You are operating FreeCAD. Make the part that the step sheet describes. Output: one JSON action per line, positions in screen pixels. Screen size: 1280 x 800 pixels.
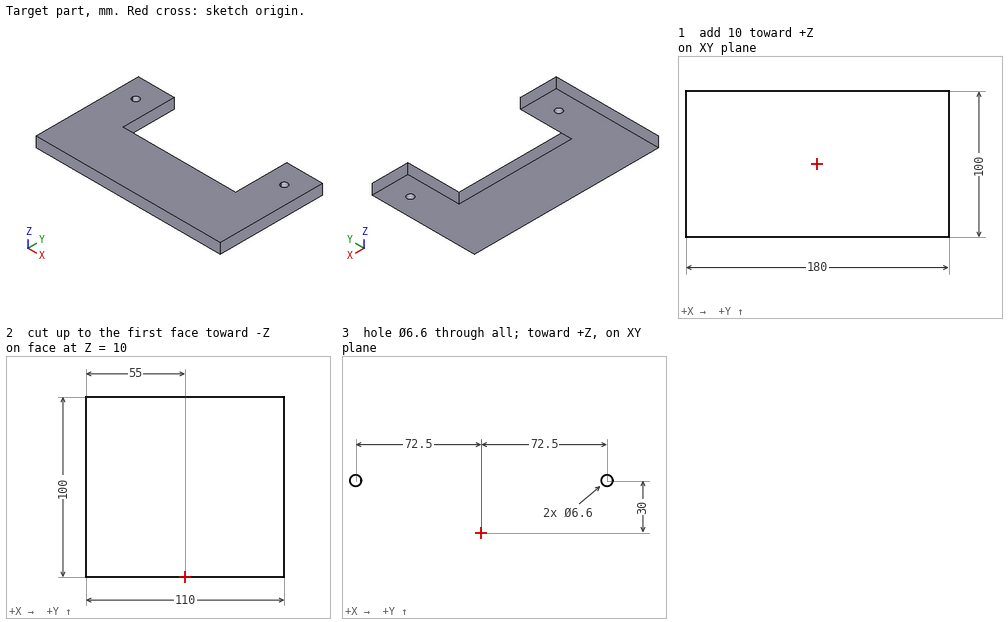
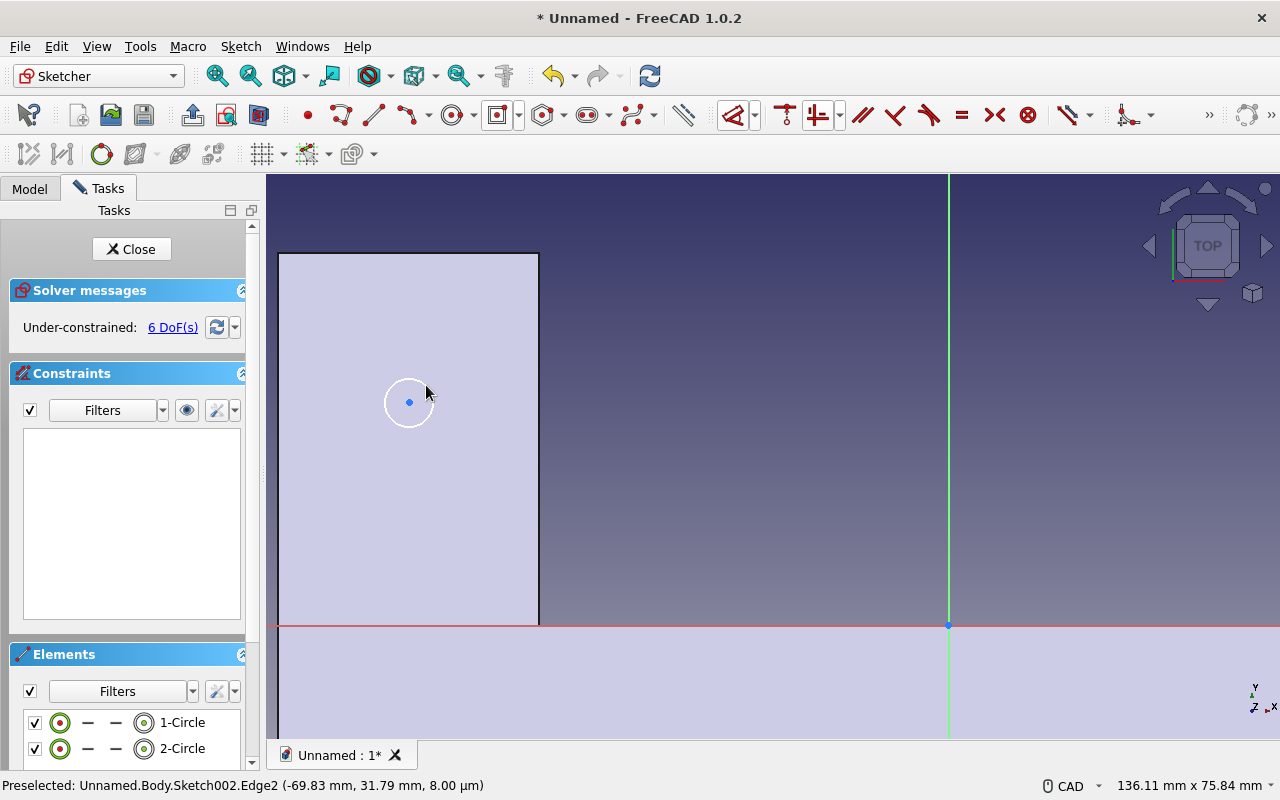
{"action": "scroll", "coordinate": [408, 402], "scroll_direction": "down", "scroll_amount": 3}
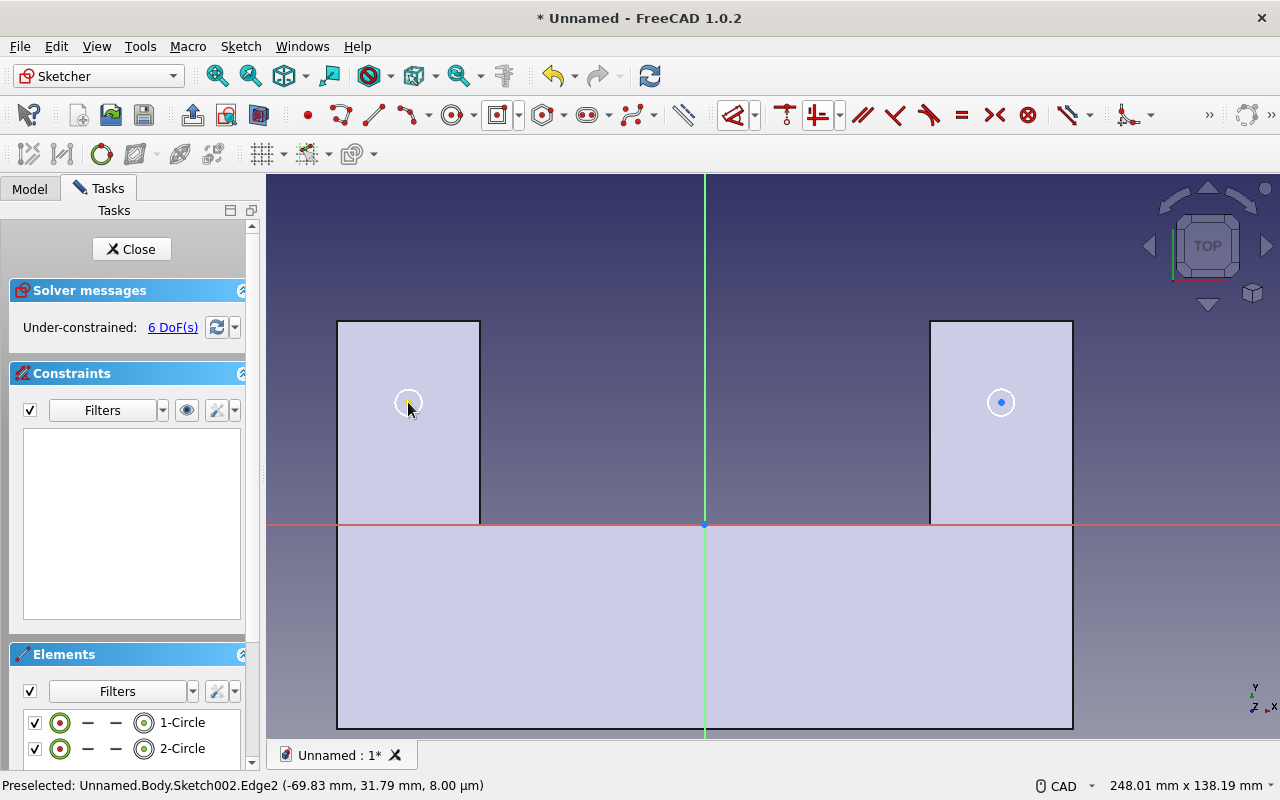
{"action": "left_click", "coordinate": [1011, 393]}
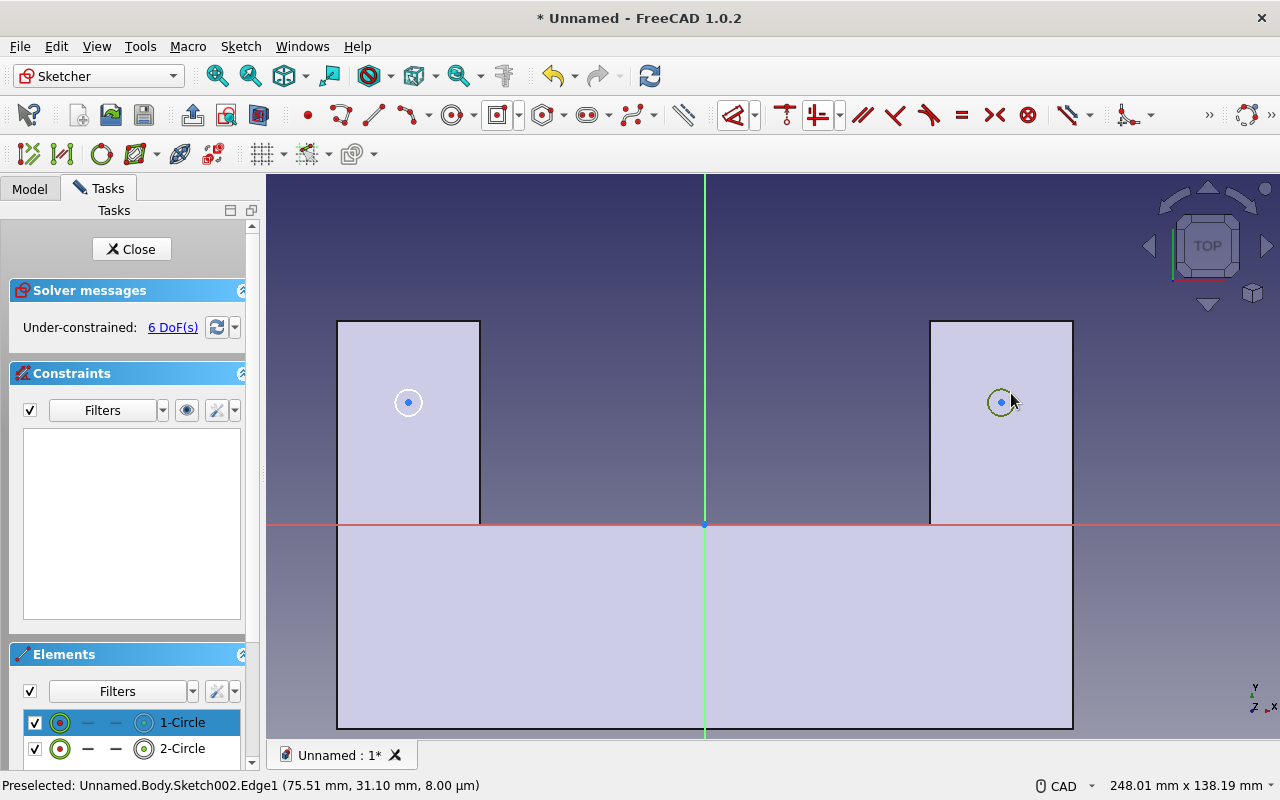
{"action": "left_click", "coordinate": [418, 393]}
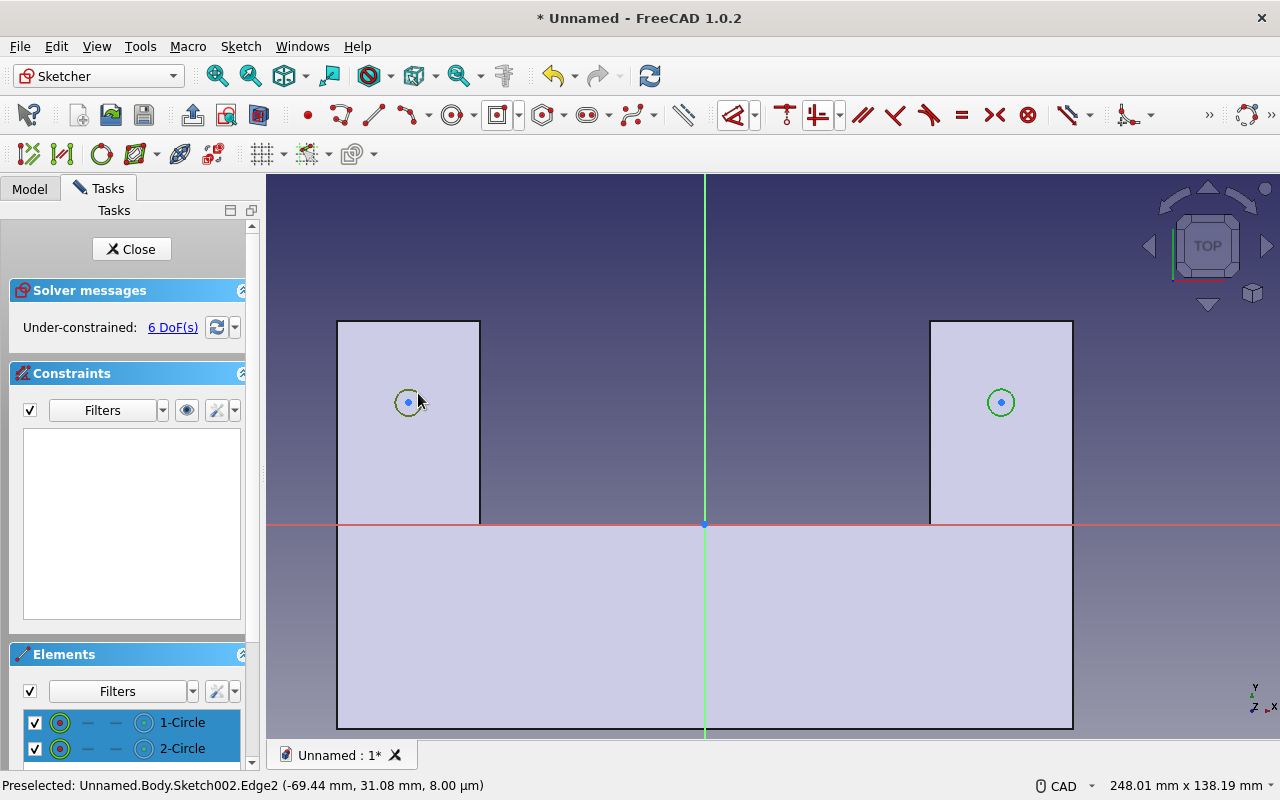
{"action": "left_click", "coordinate": [962, 116]}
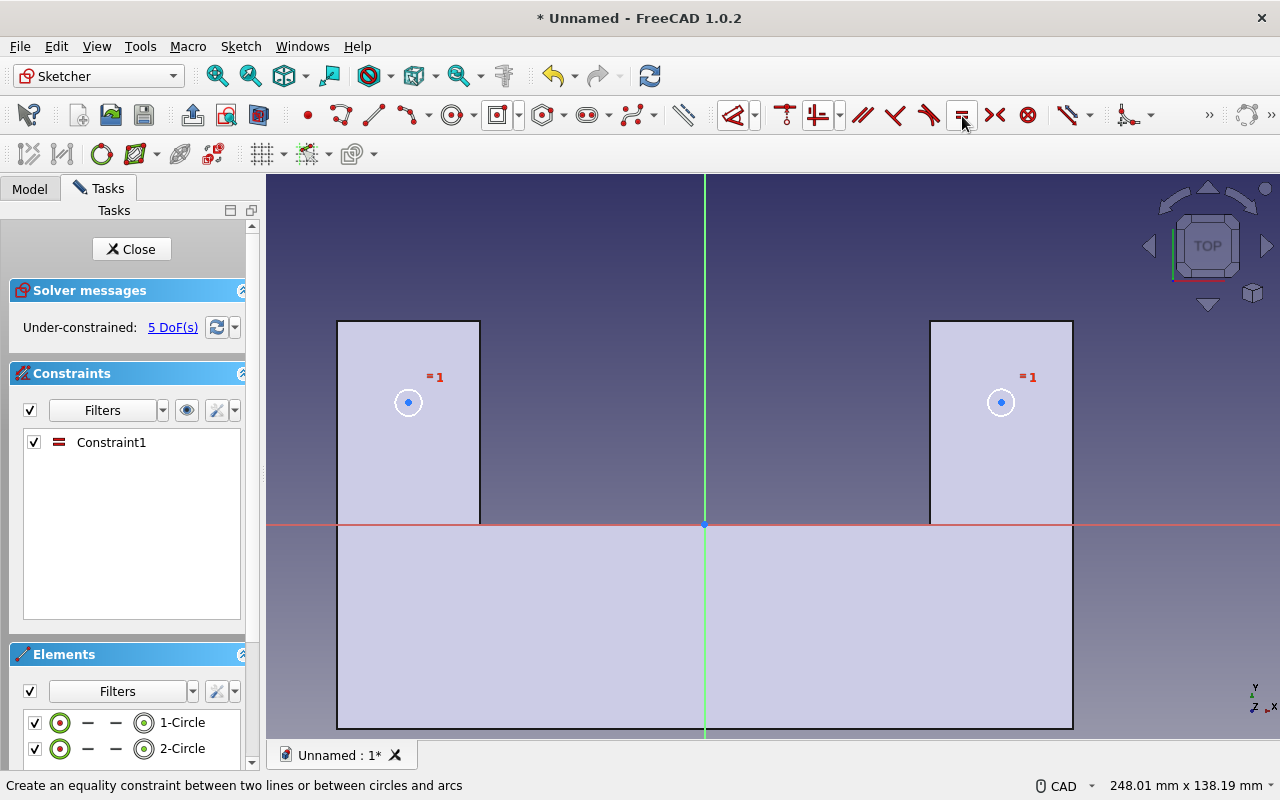
{"action": "left_click", "coordinate": [1001, 403]}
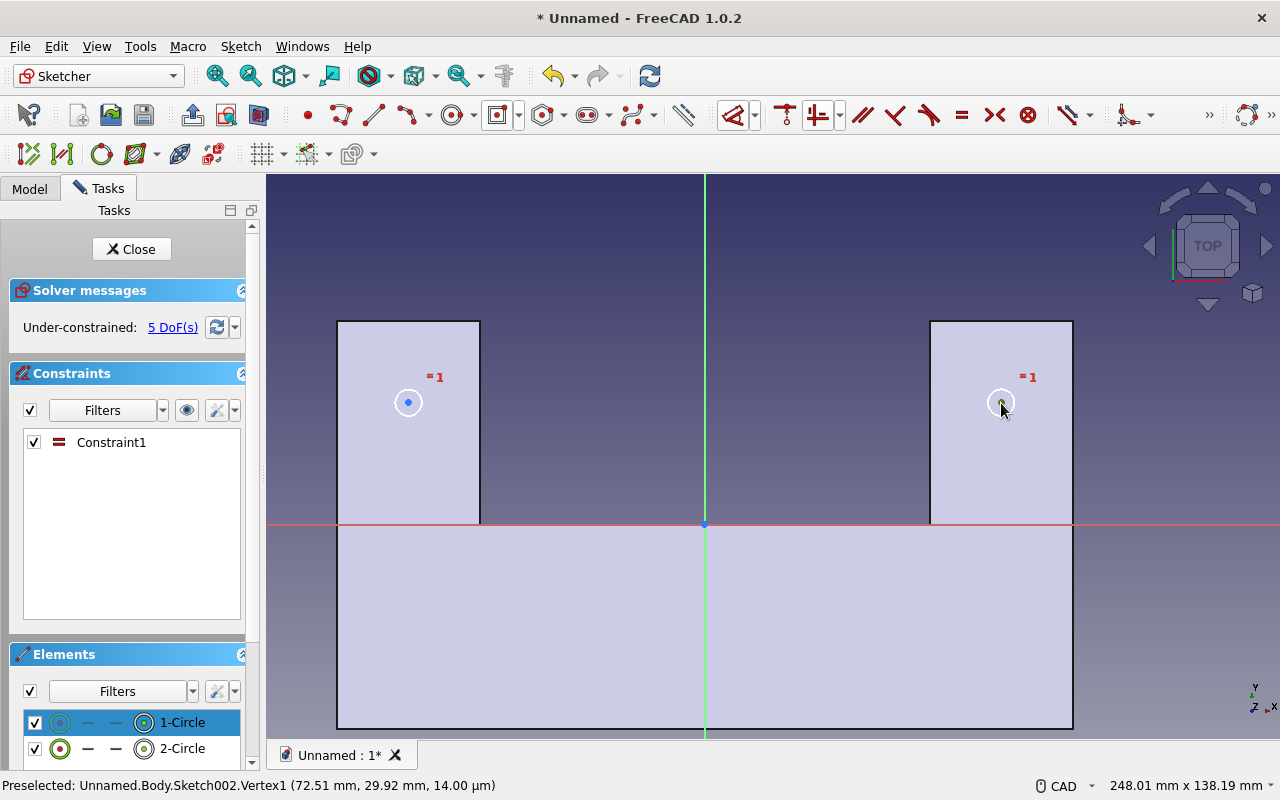
{"action": "left_click", "coordinate": [409, 403]}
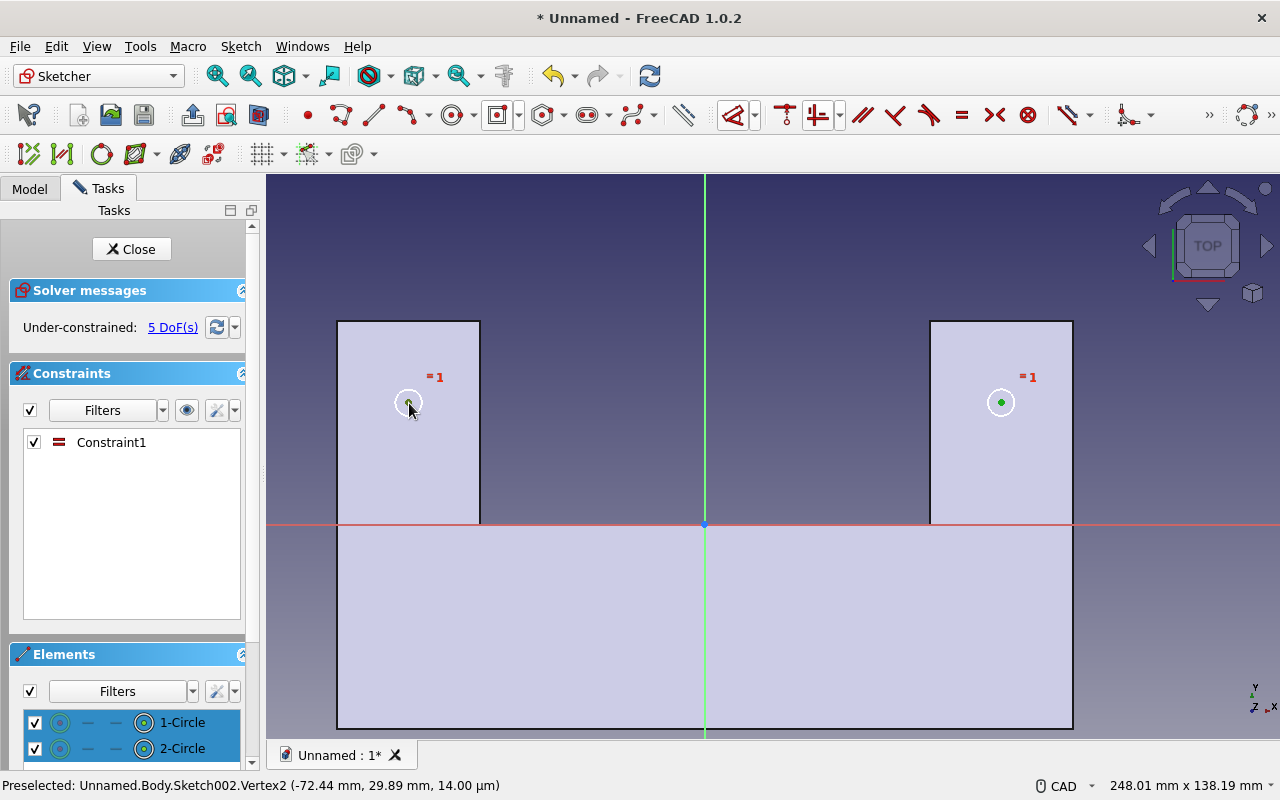
{"action": "key", "text": "h"}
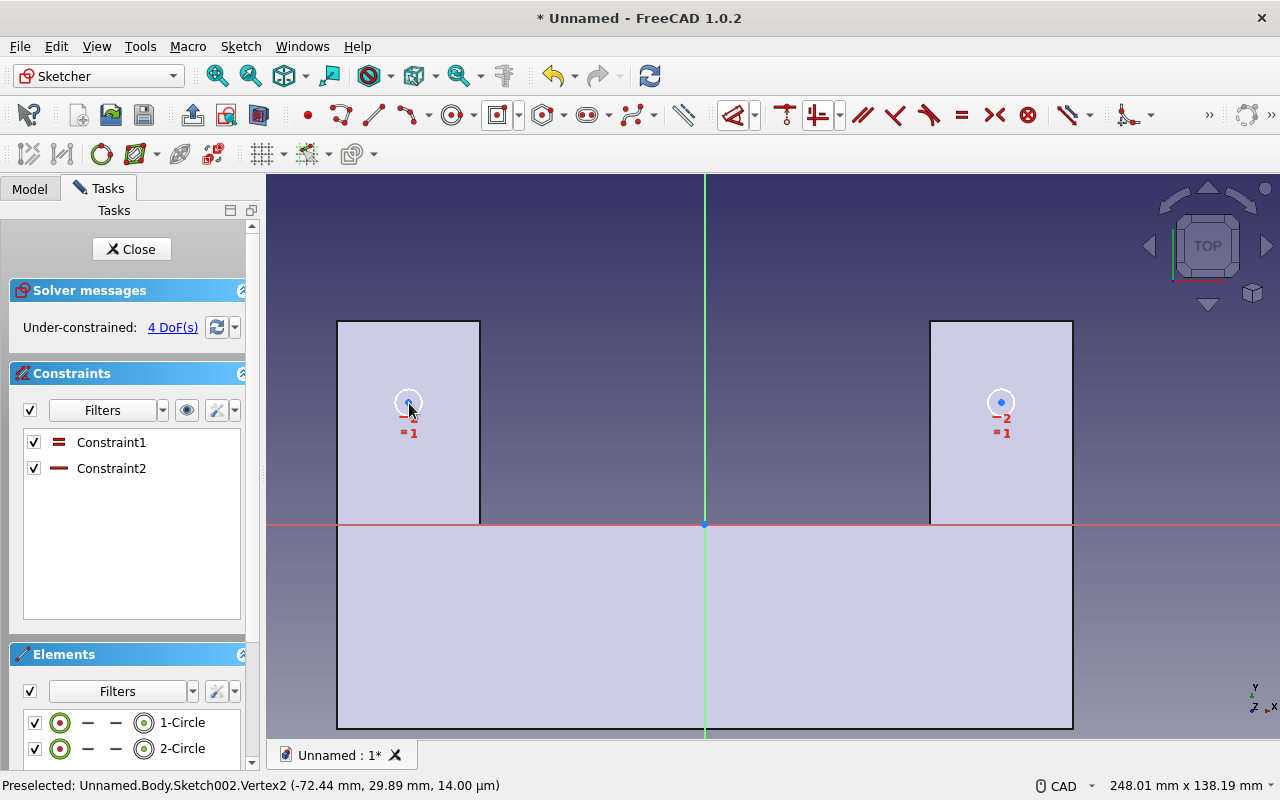
{"action": "scroll", "coordinate": [1011, 393], "scroll_direction": "up", "scroll_amount": 2}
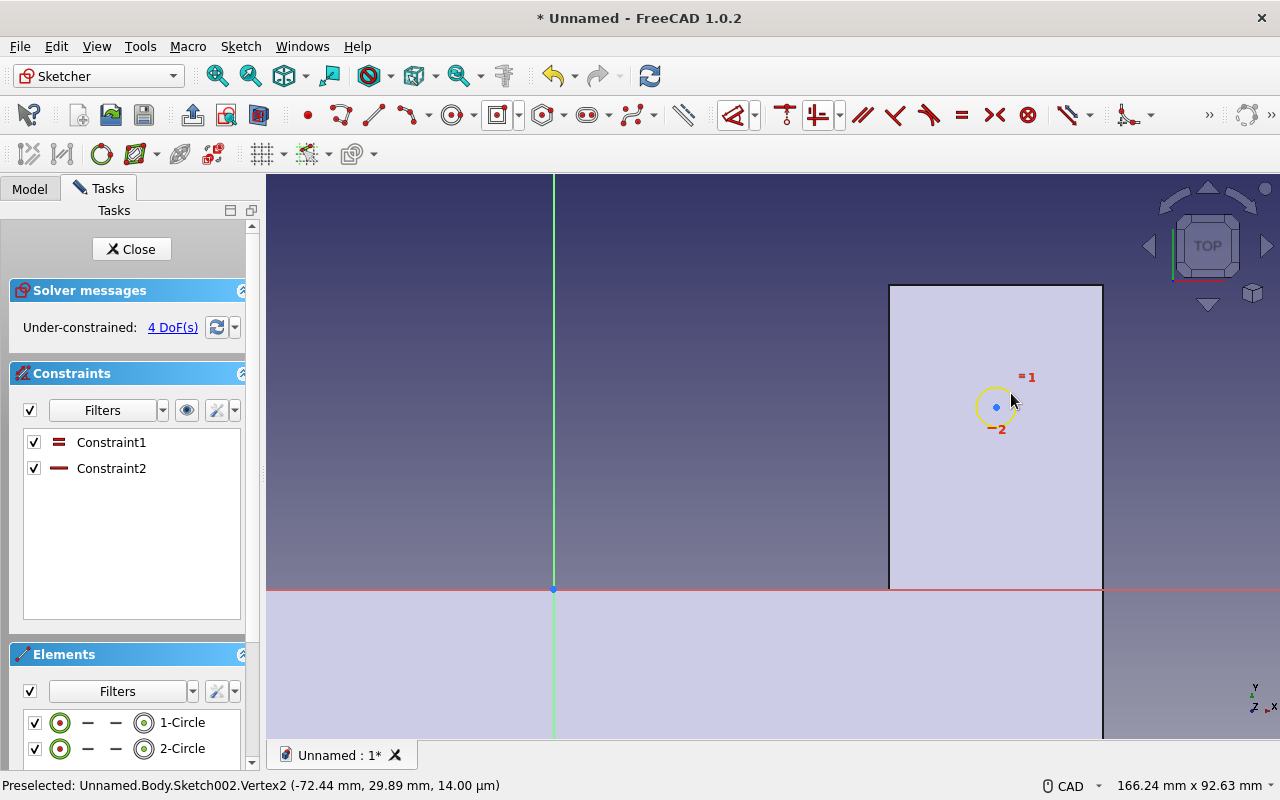
{"action": "left_click", "coordinate": [1010, 393]}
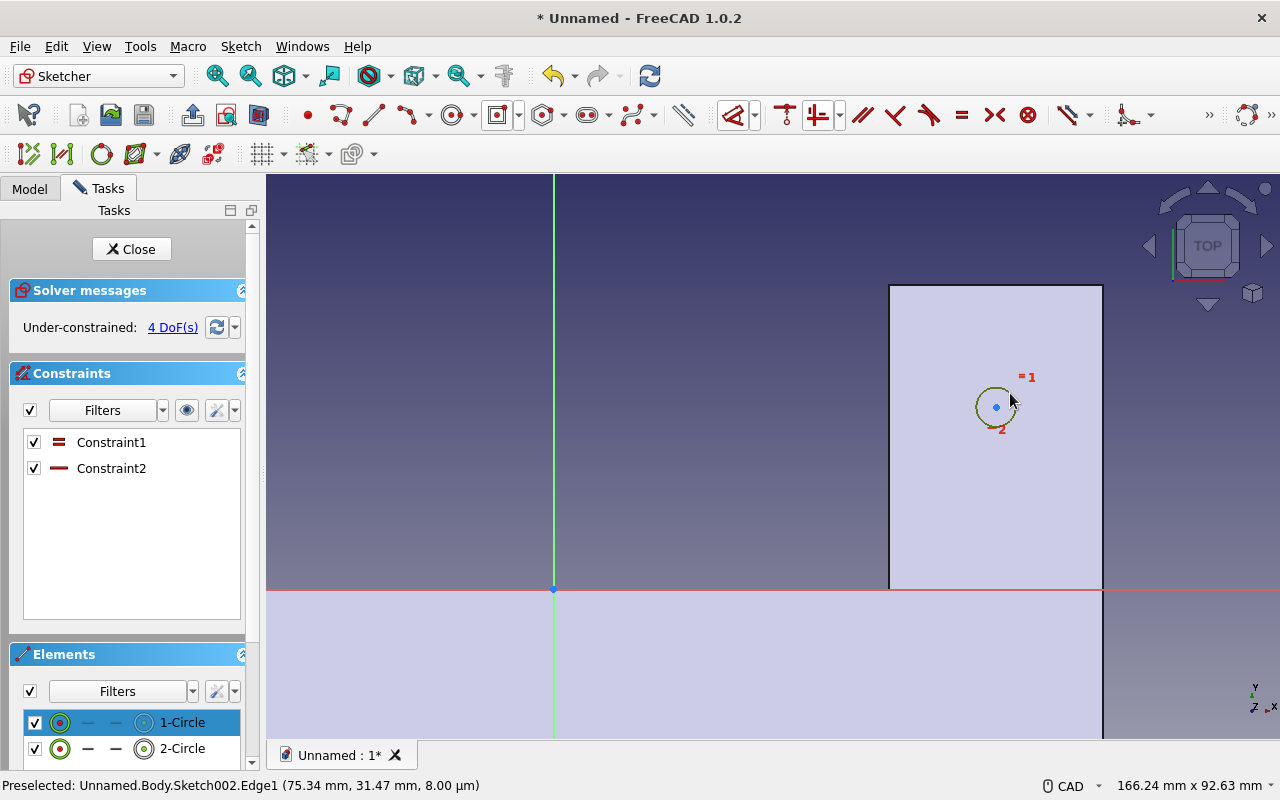
{"action": "left_click", "coordinate": [754, 116]}